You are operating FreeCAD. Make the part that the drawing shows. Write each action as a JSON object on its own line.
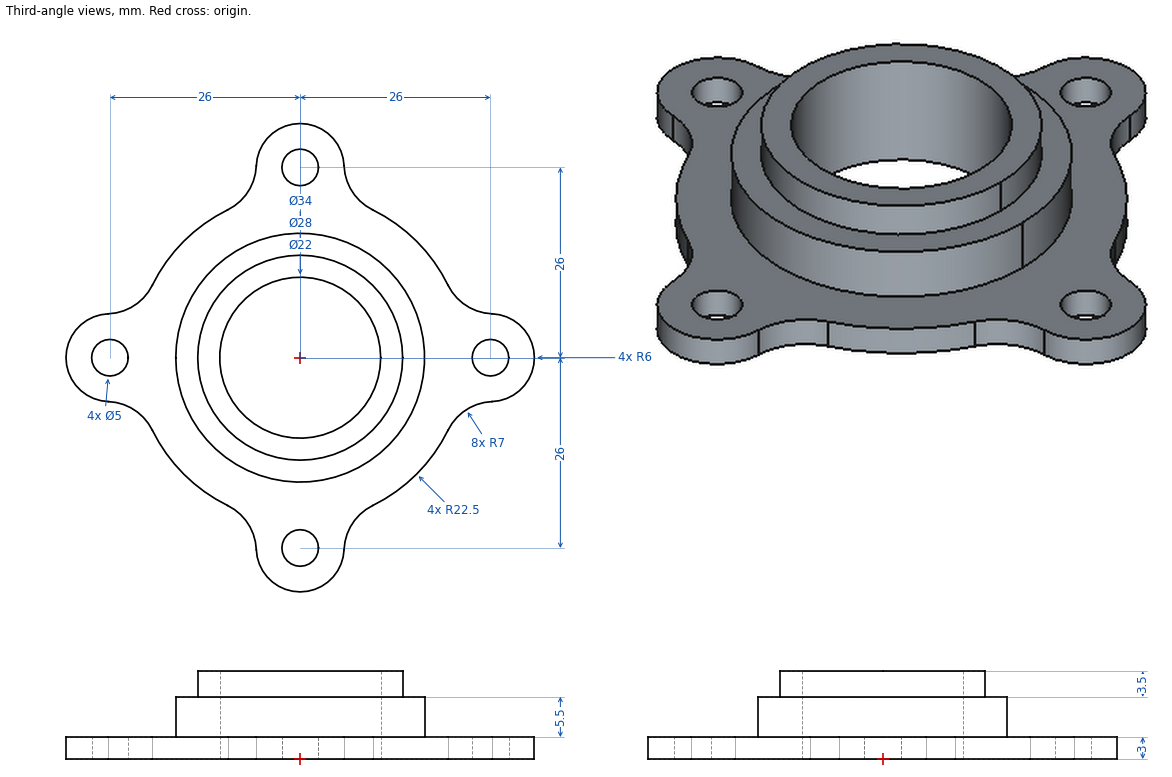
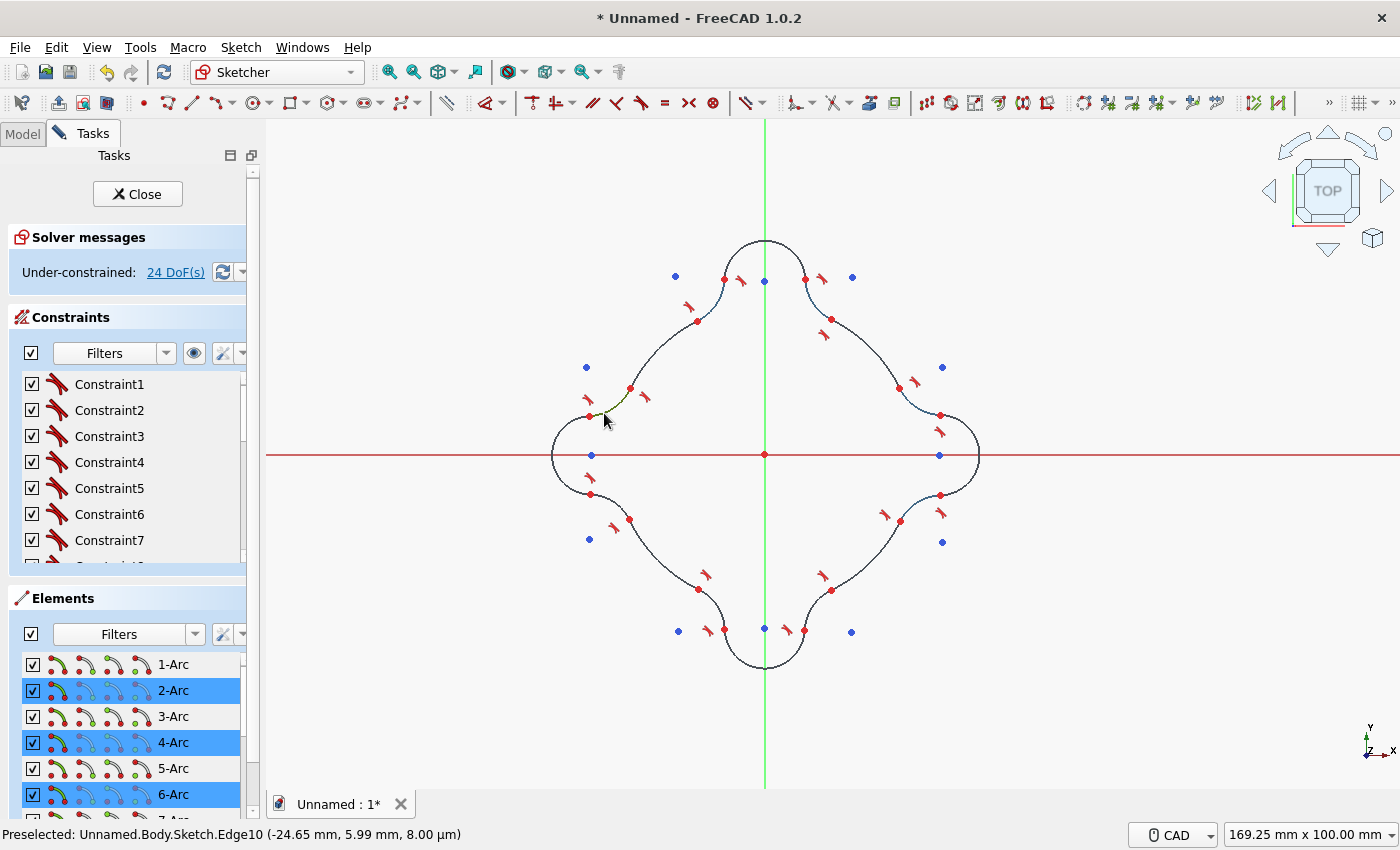
{"action": "left_click", "coordinate": [621, 508]}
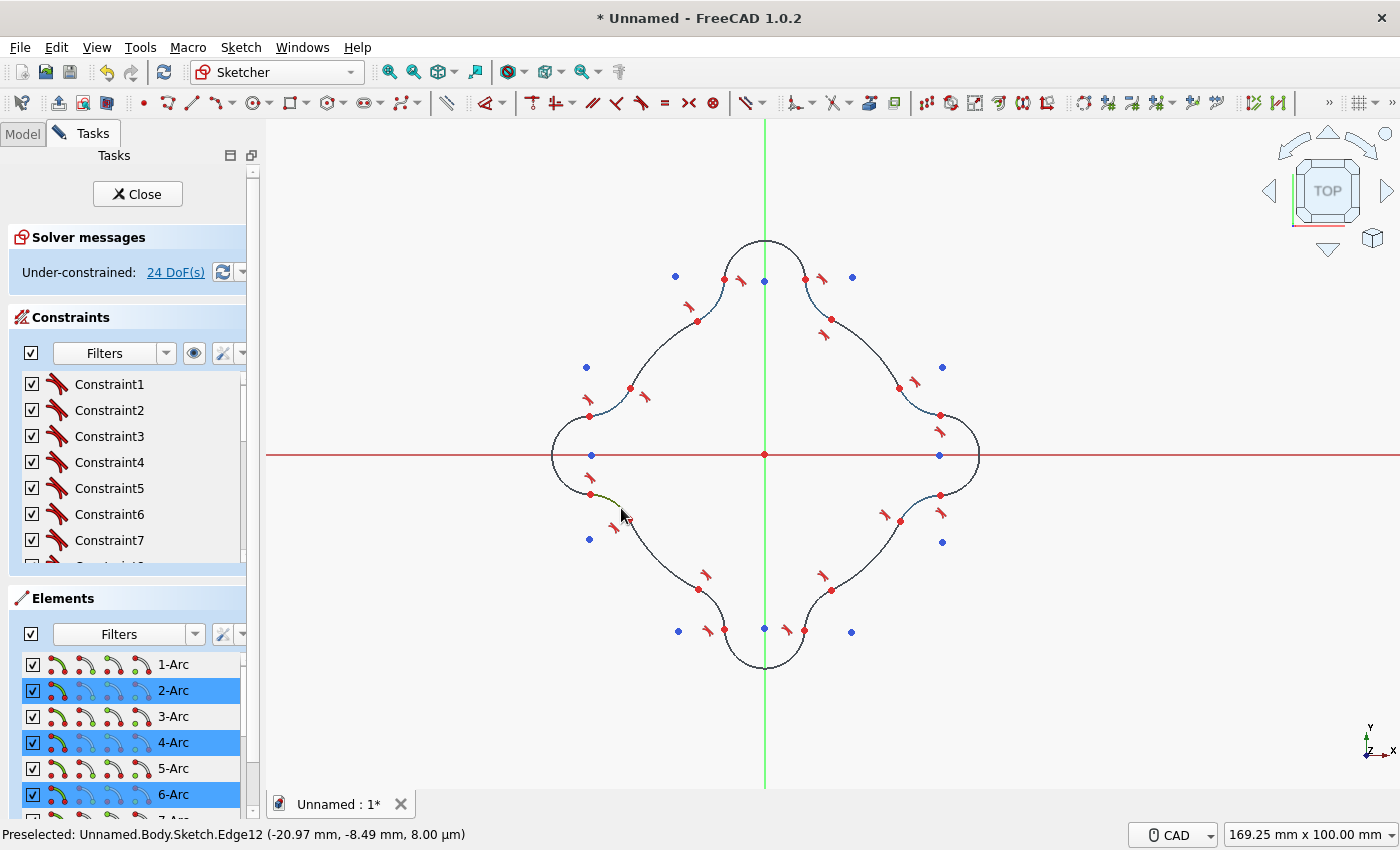
{"action": "left_click", "coordinate": [722, 615]}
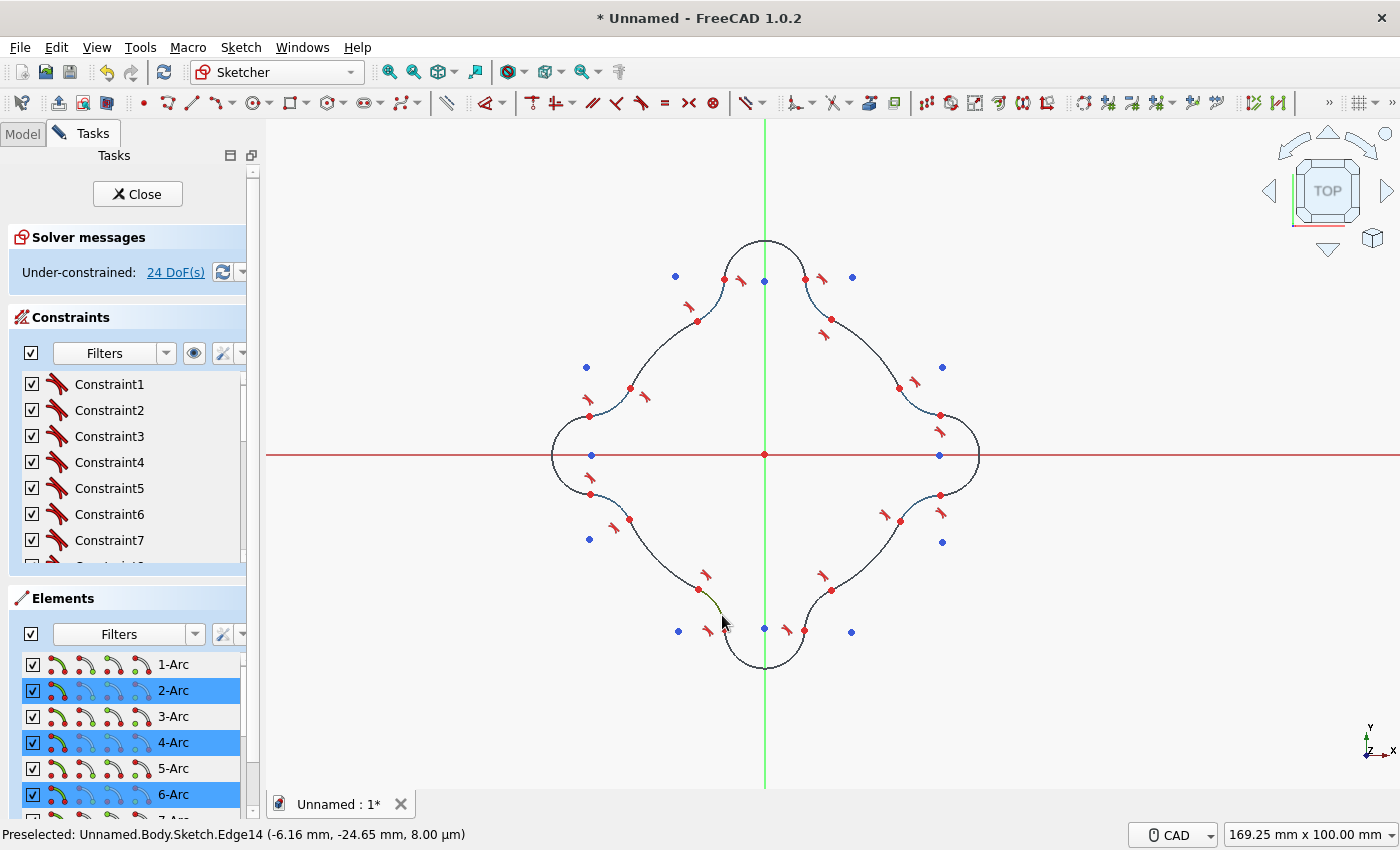
{"action": "left_click", "coordinate": [819, 599]}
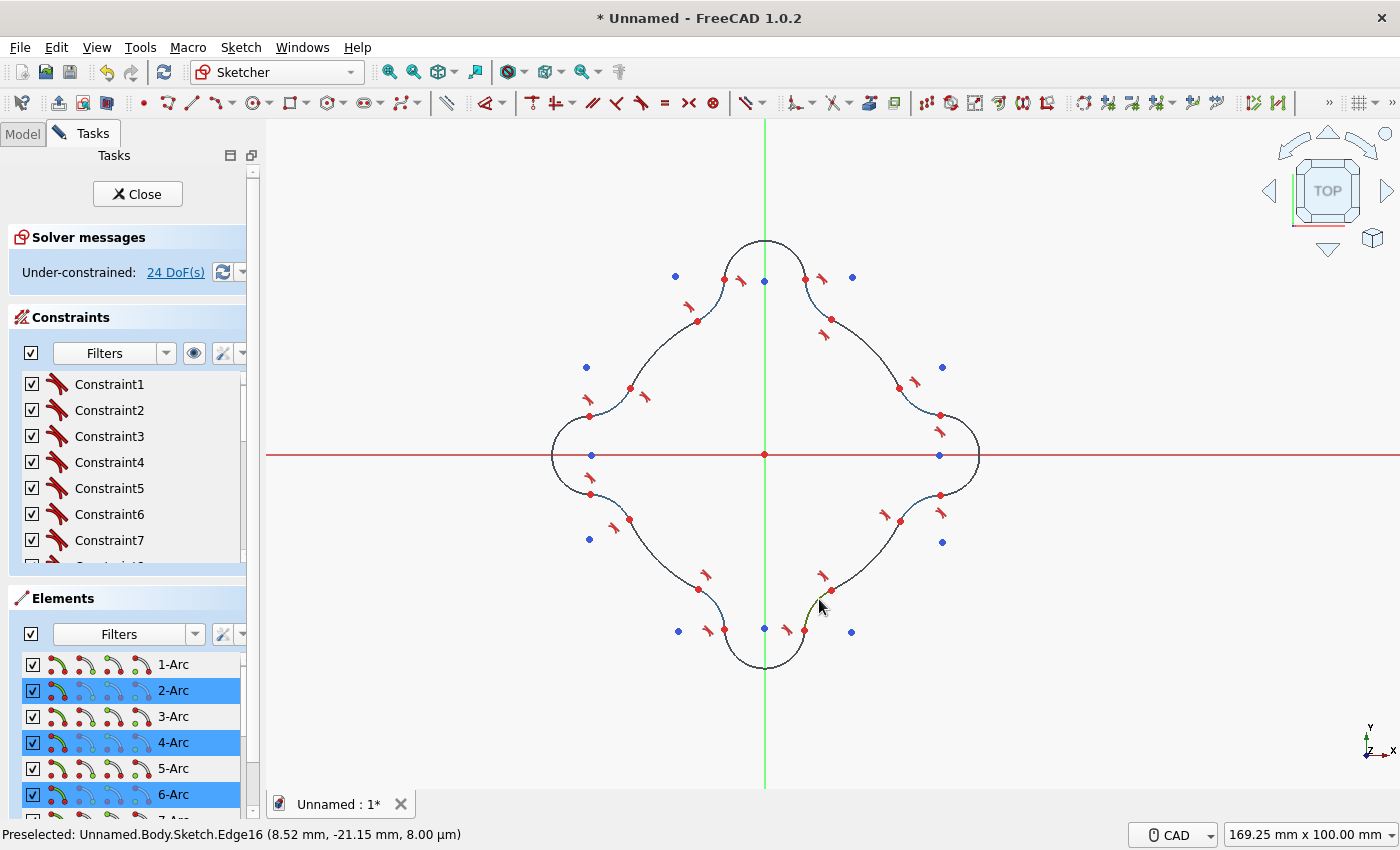
{"action": "left_click", "coordinate": [666, 104]}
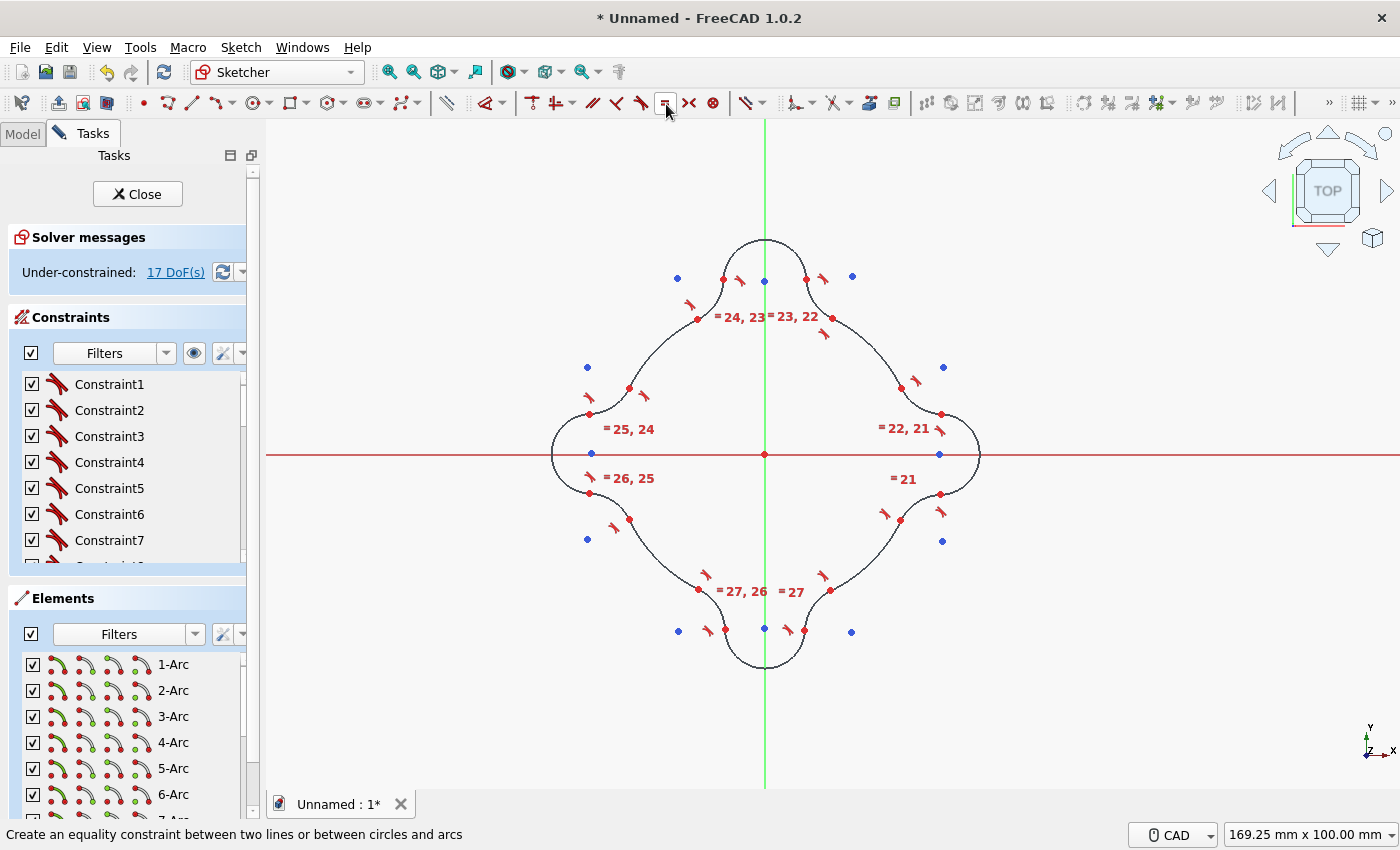
{"action": "left_click", "coordinate": [857, 575]}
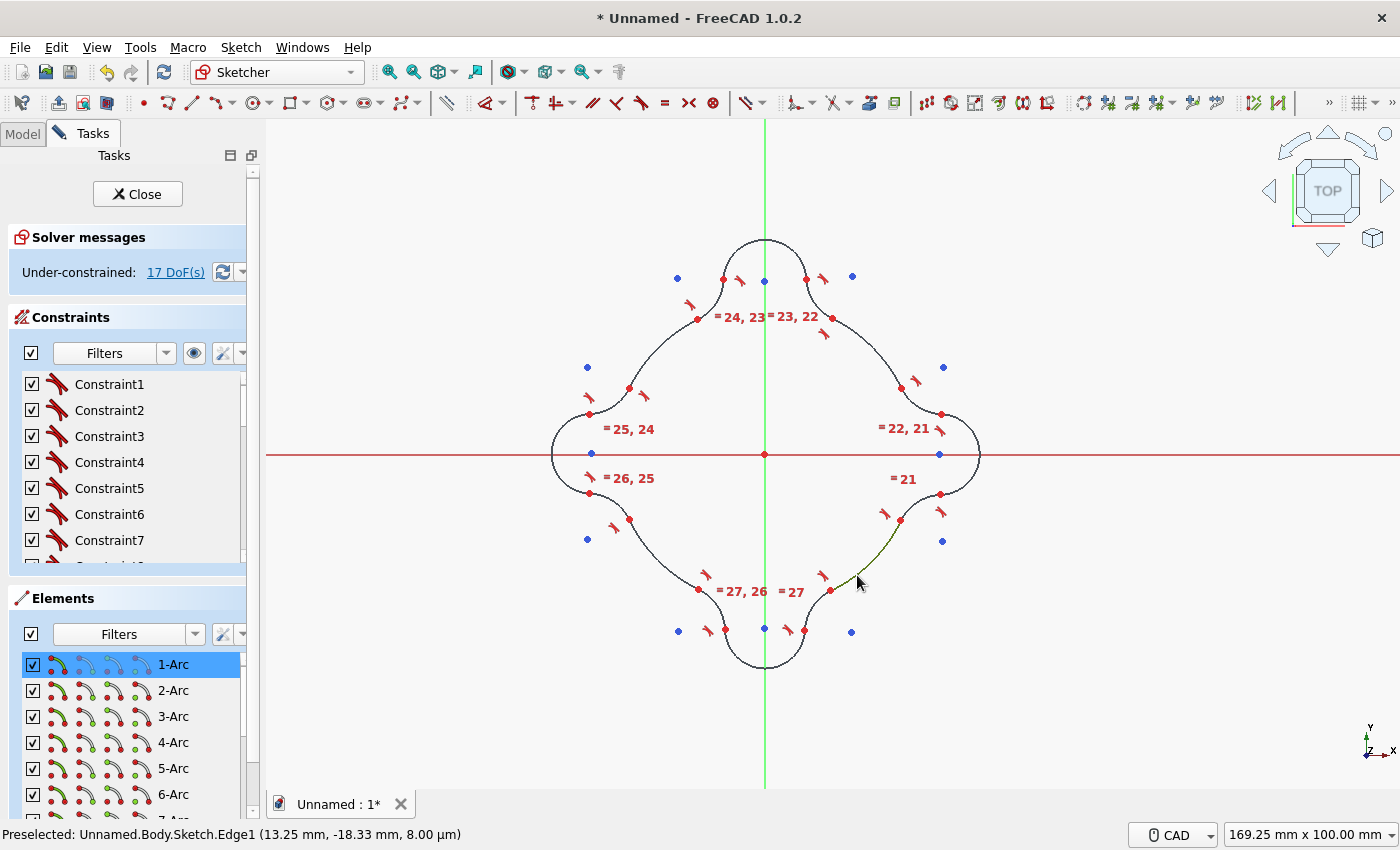
{"action": "left_click", "coordinate": [886, 363]}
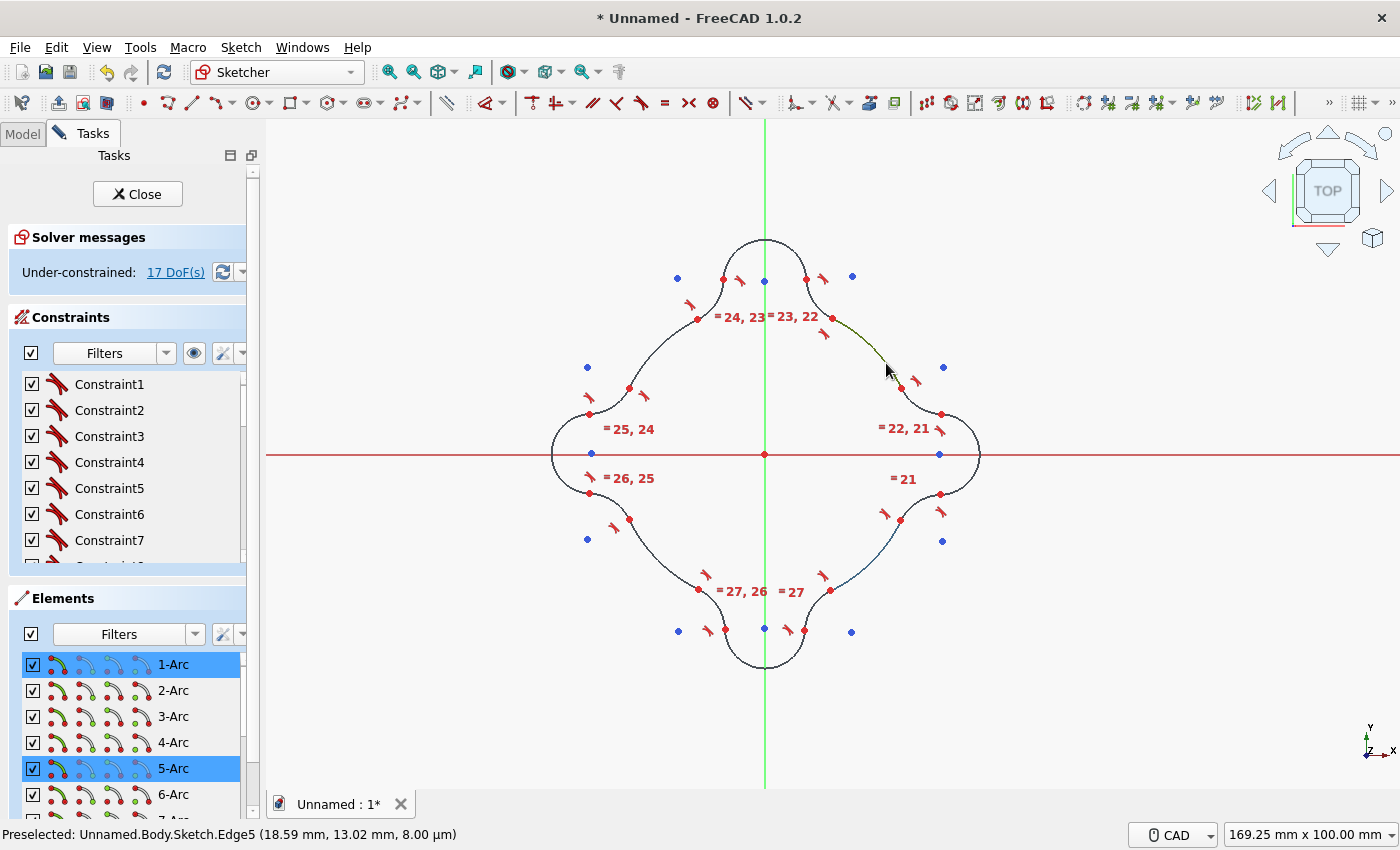
{"action": "left_click", "coordinate": [673, 335]}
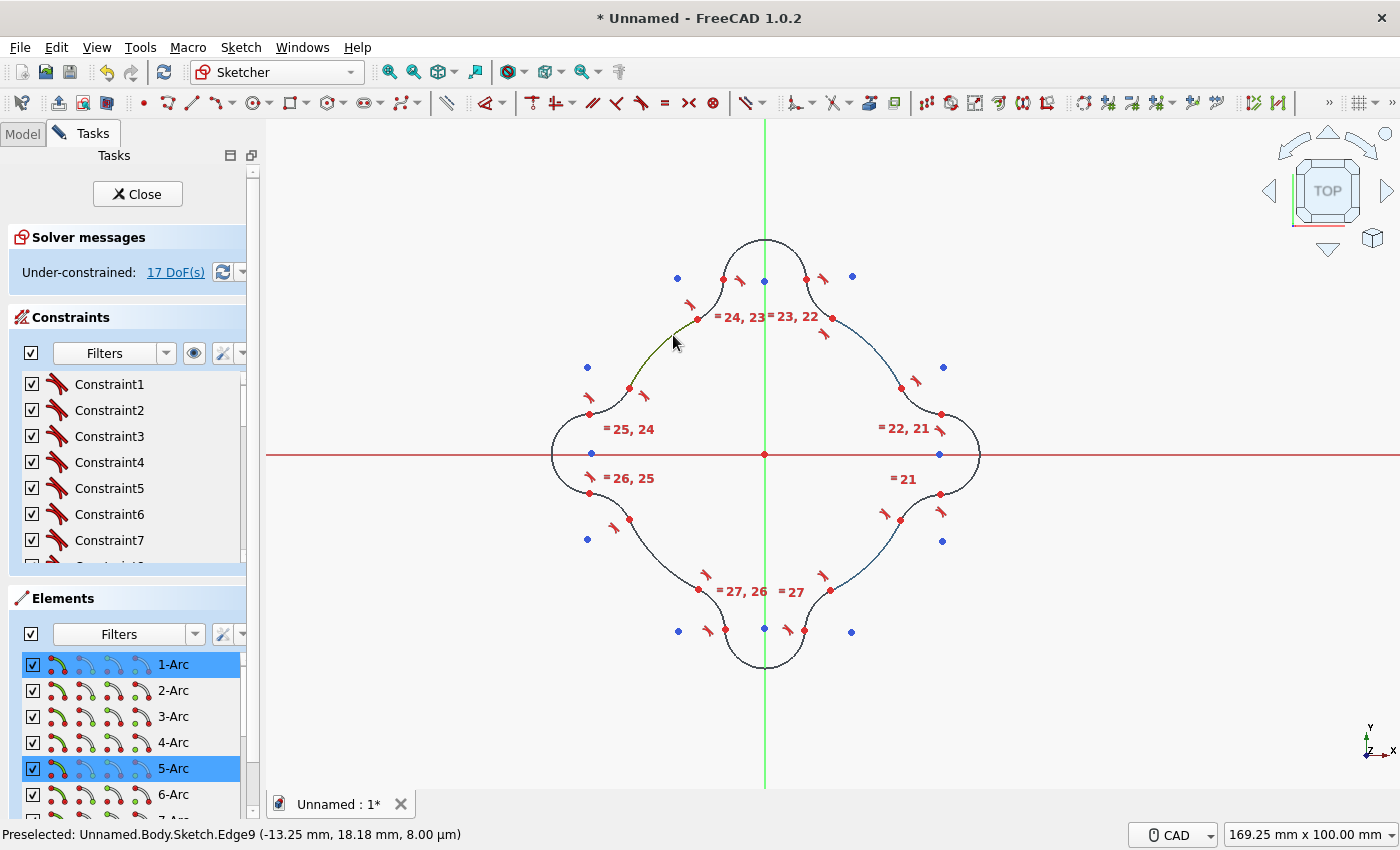
{"action": "left_click", "coordinate": [645, 545]}